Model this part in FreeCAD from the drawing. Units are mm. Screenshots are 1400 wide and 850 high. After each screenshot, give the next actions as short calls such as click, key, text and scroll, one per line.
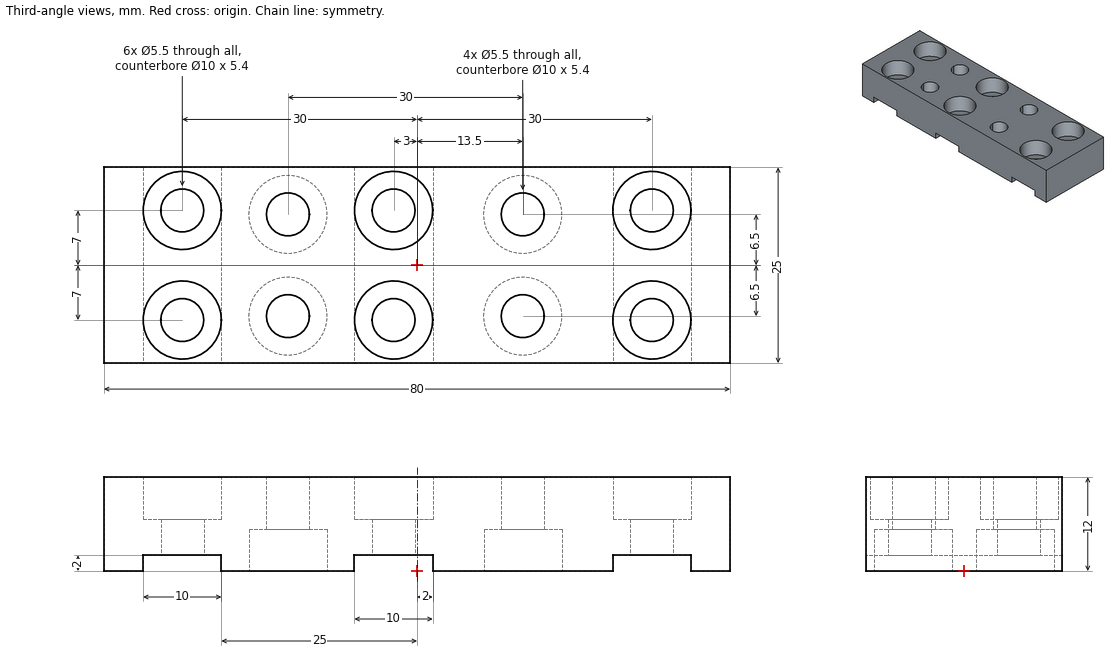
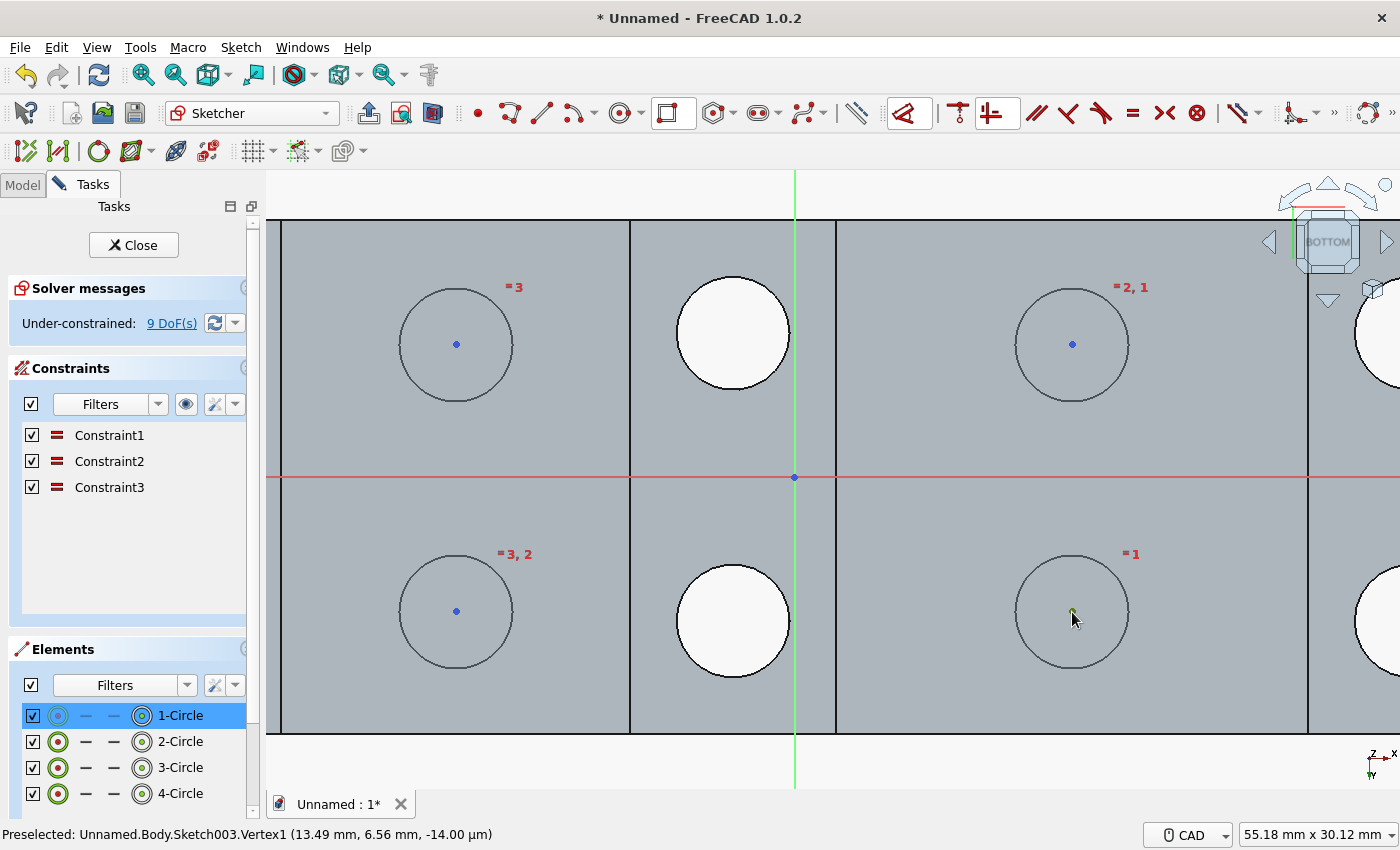
click(1072, 345)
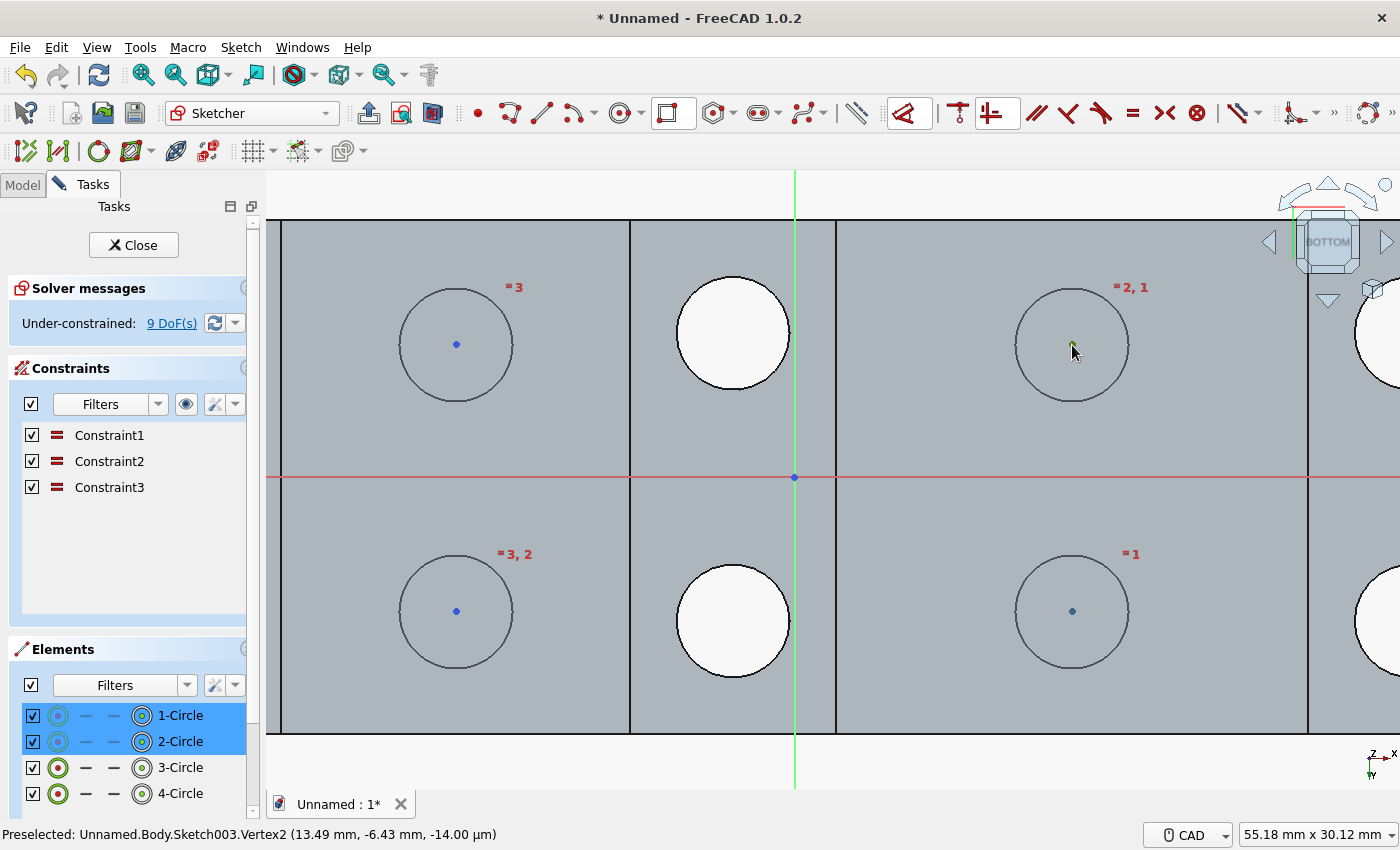
key(v)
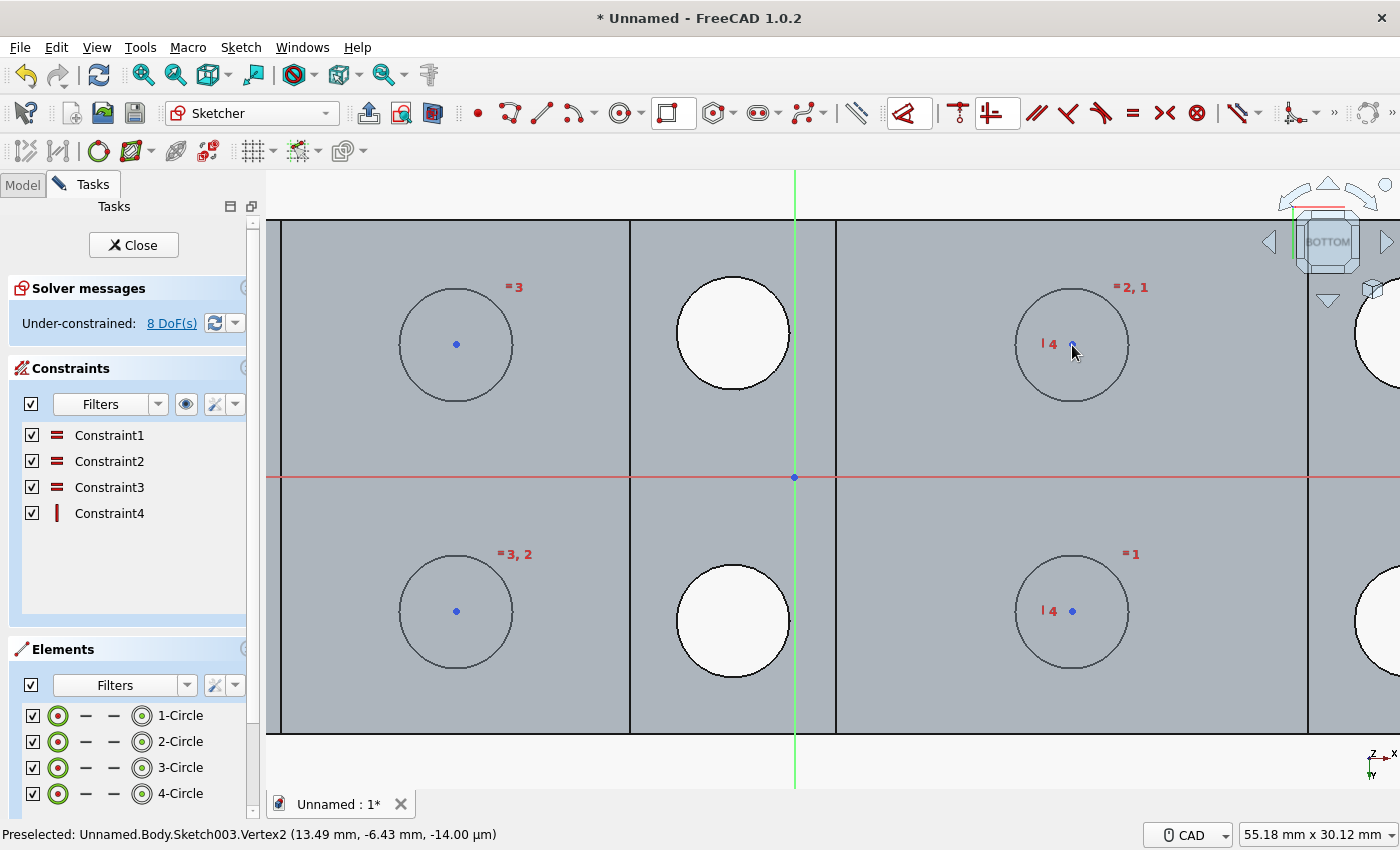
click(1072, 612)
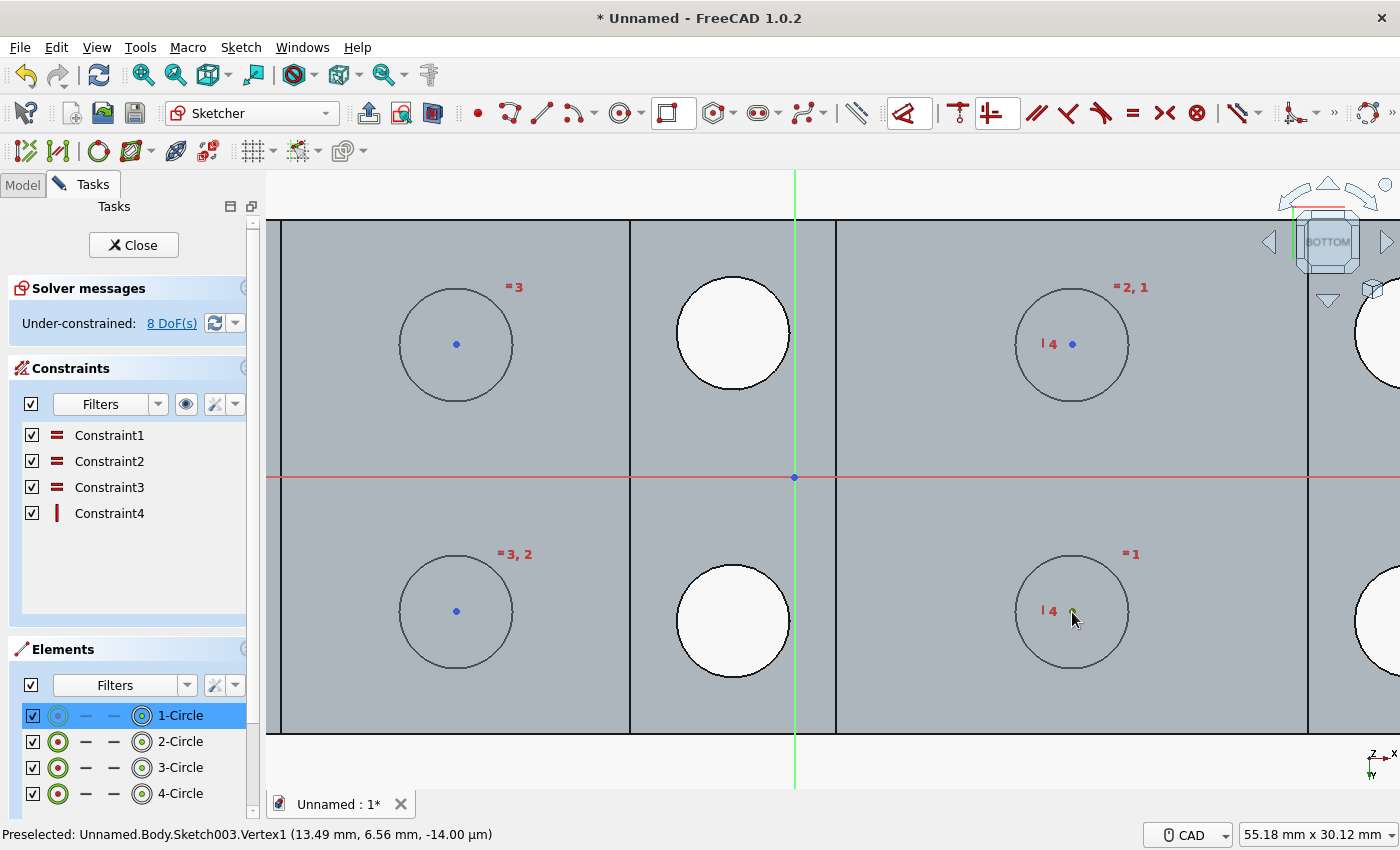
click(456, 612)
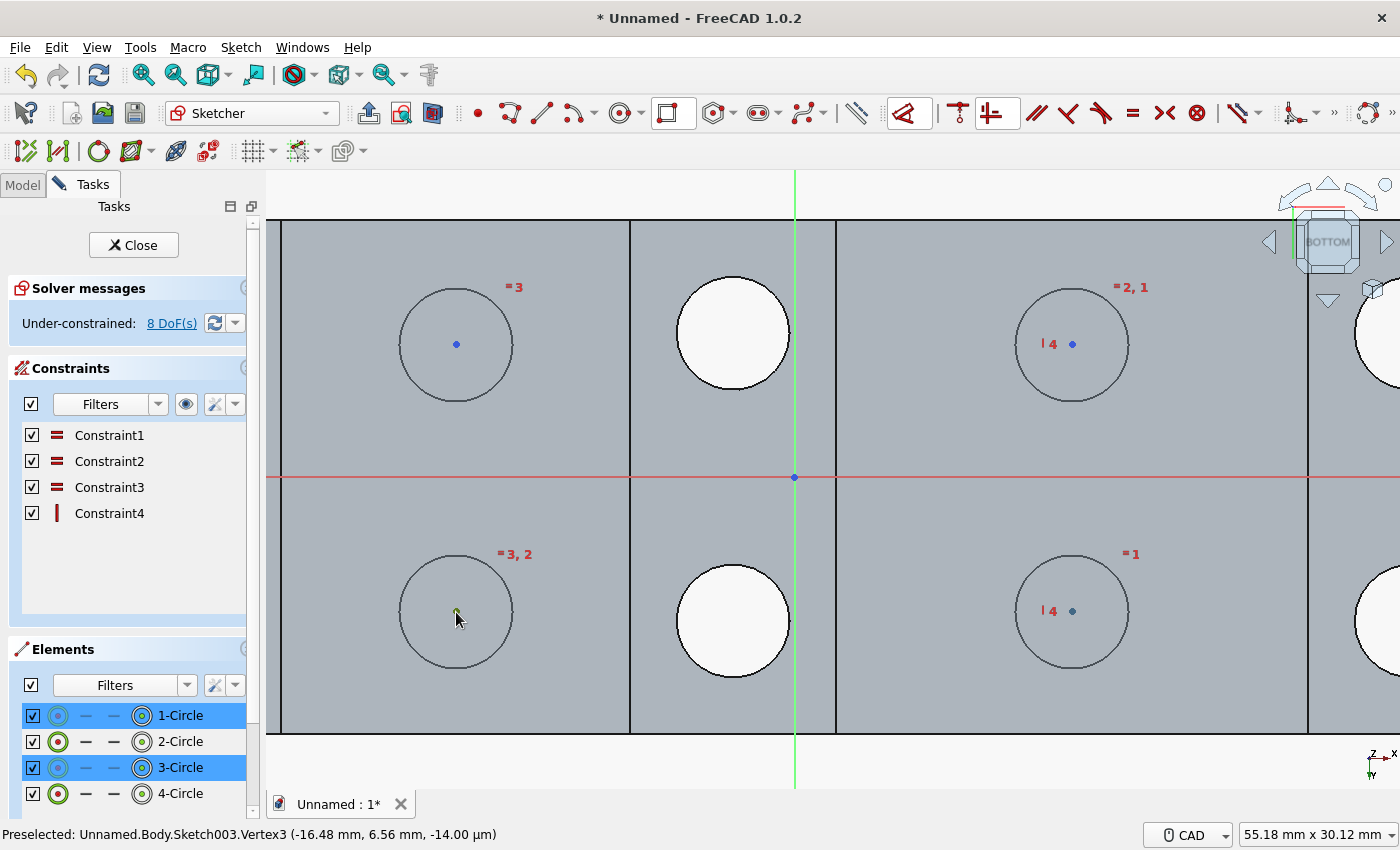
key(h)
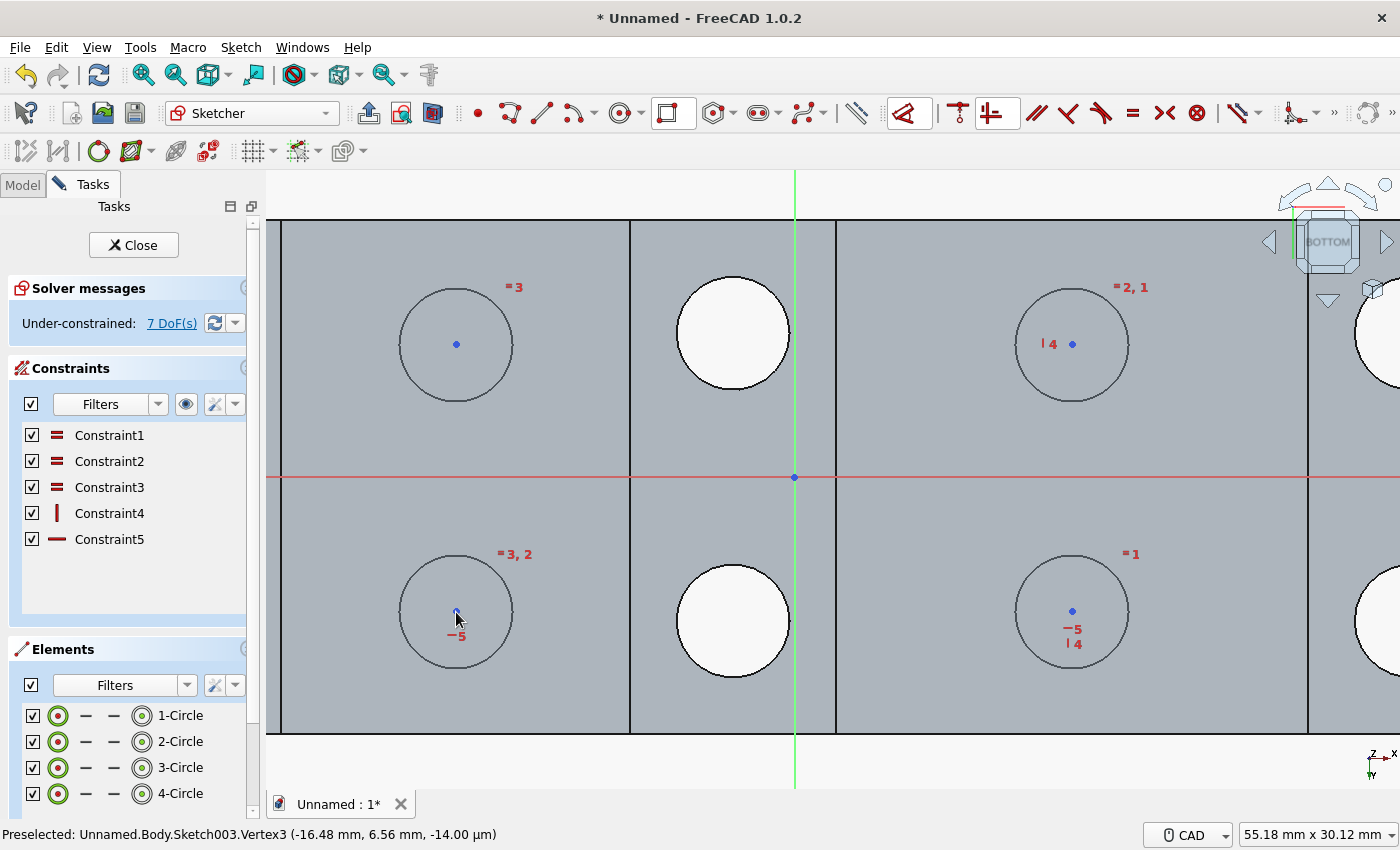
click(456, 612)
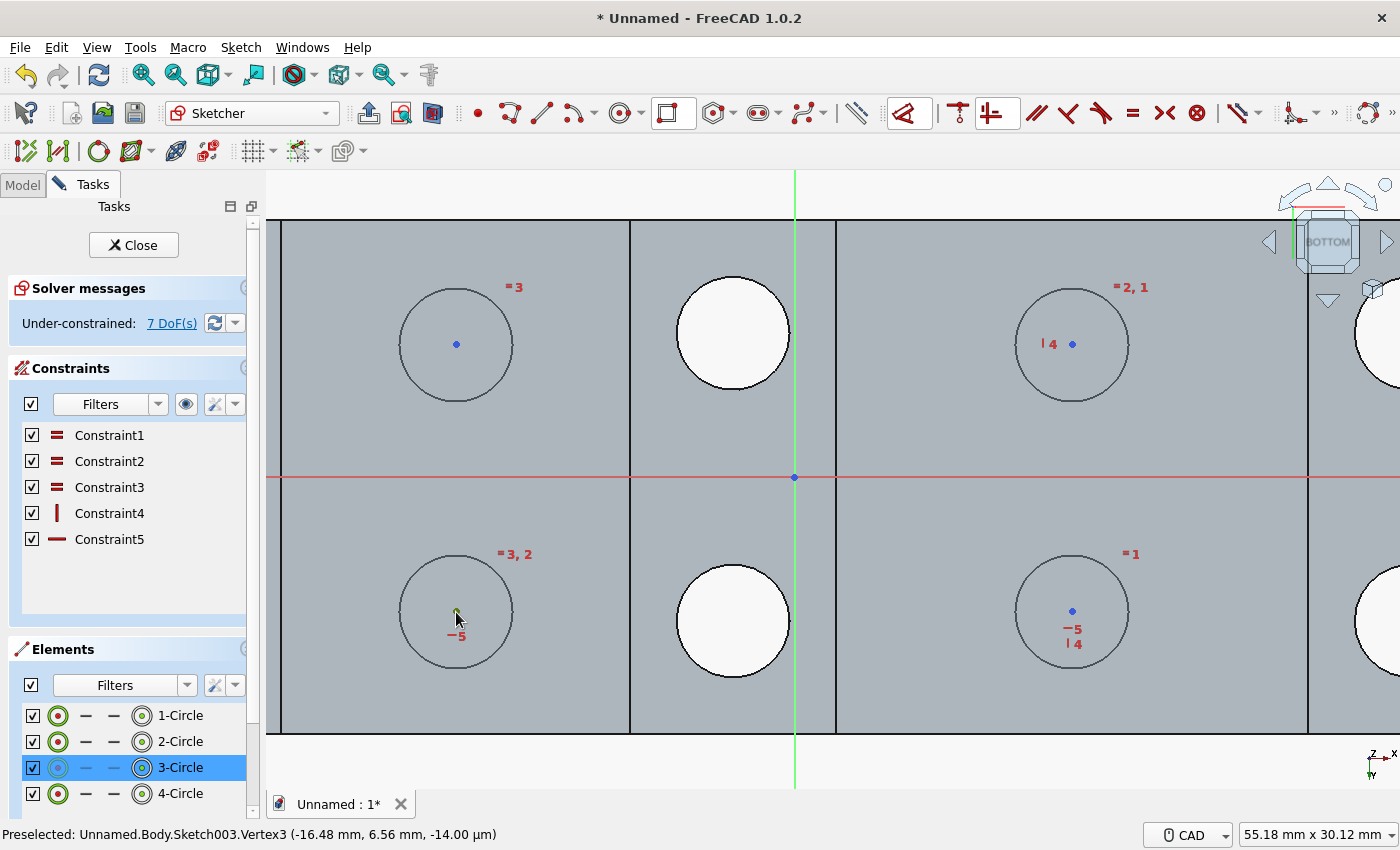
click(456, 345)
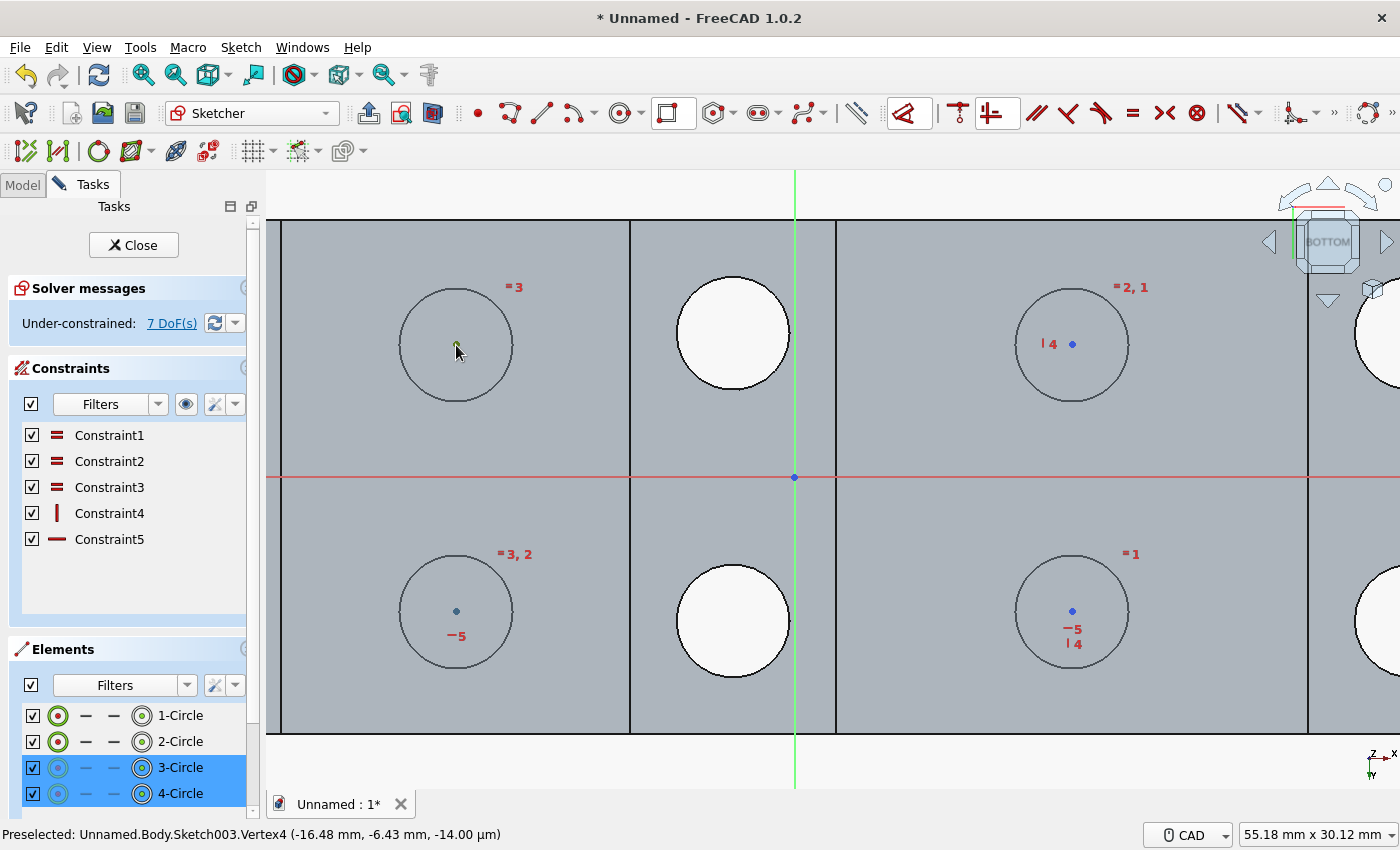
click(1014, 114)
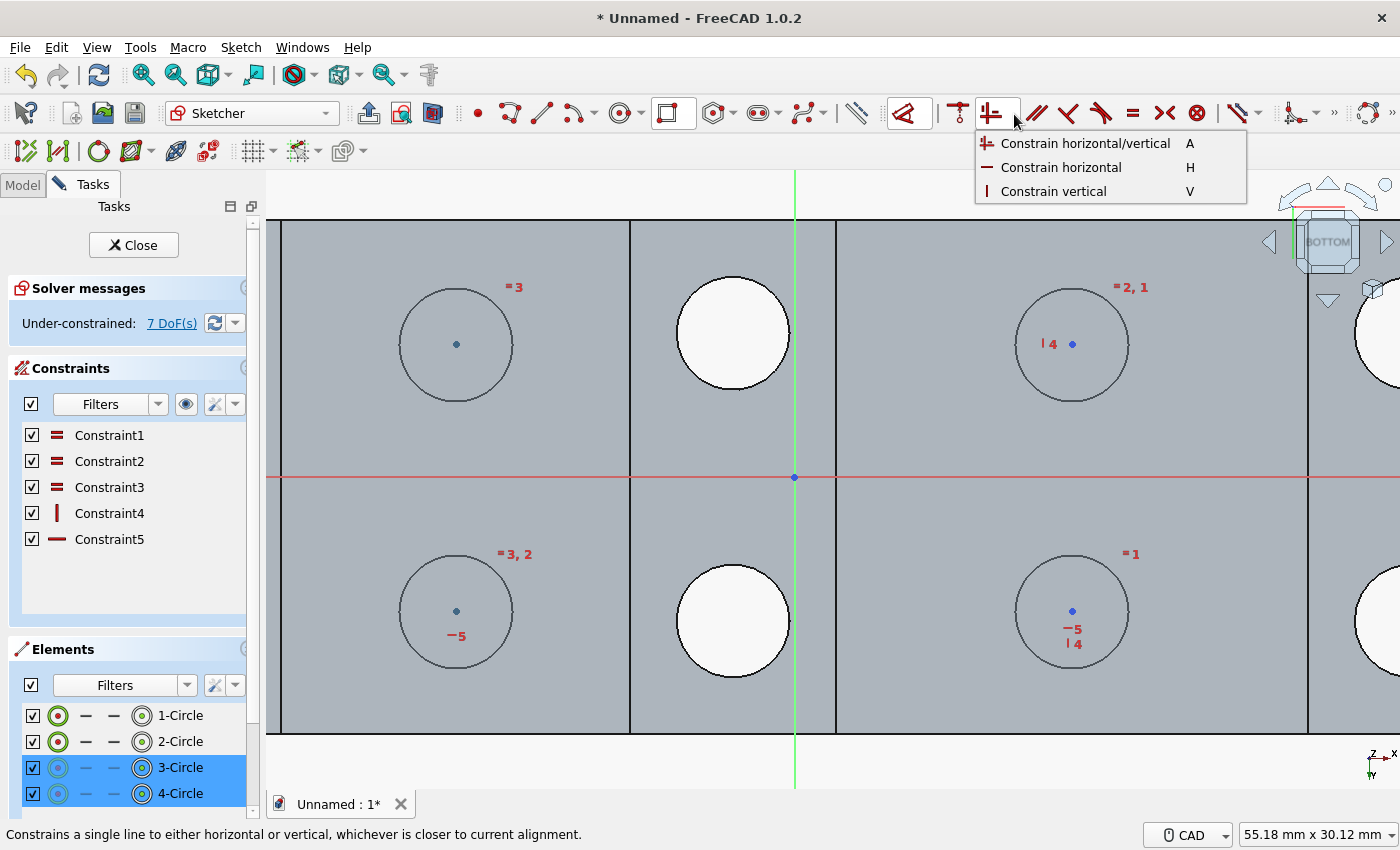
click(1111, 191)